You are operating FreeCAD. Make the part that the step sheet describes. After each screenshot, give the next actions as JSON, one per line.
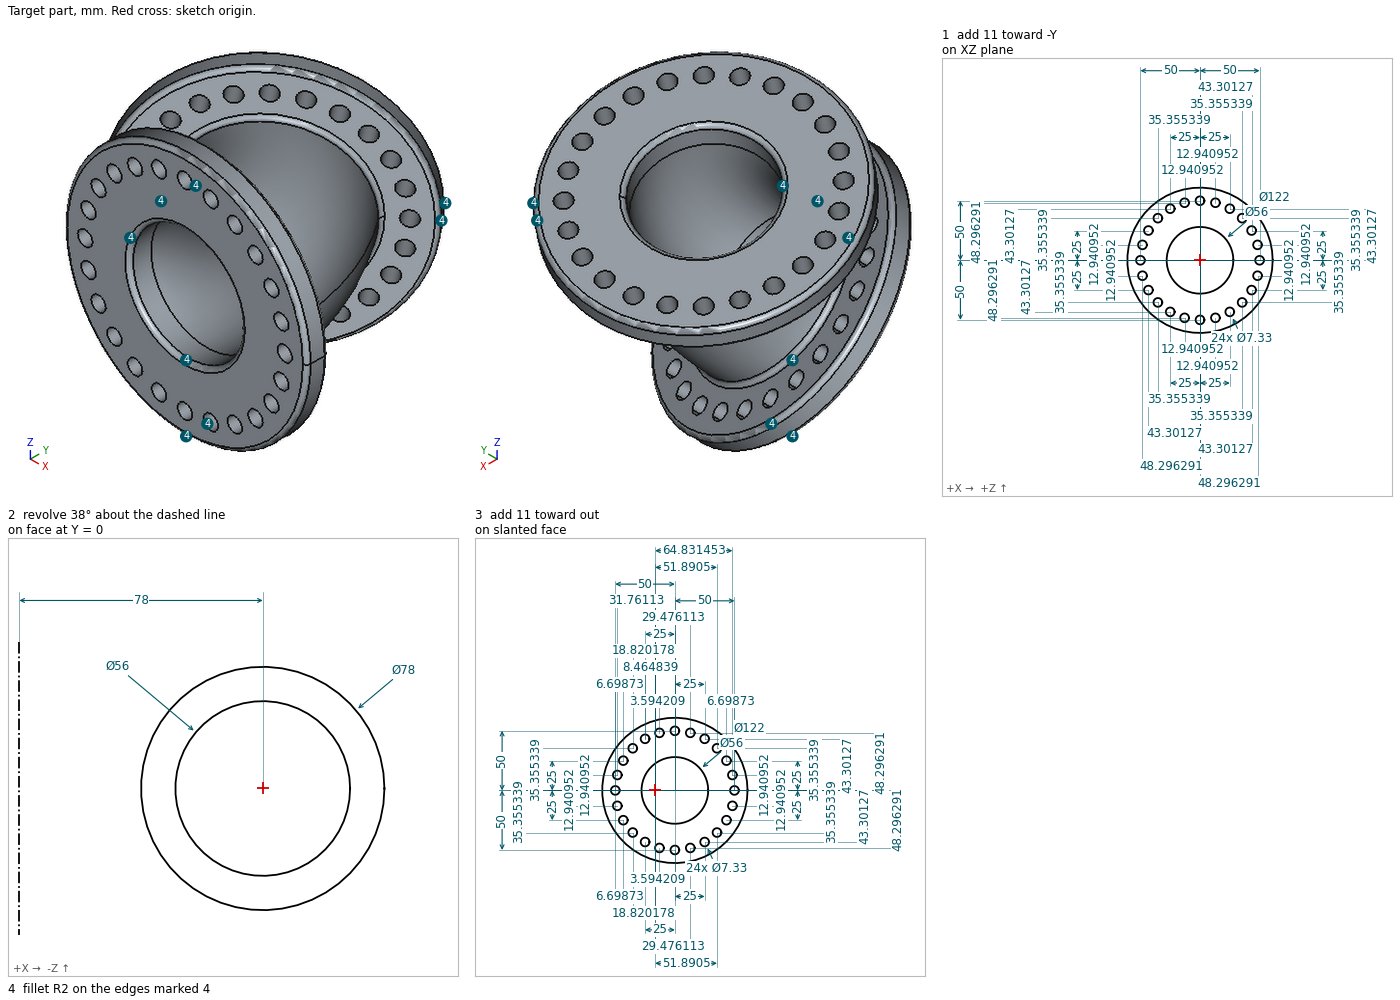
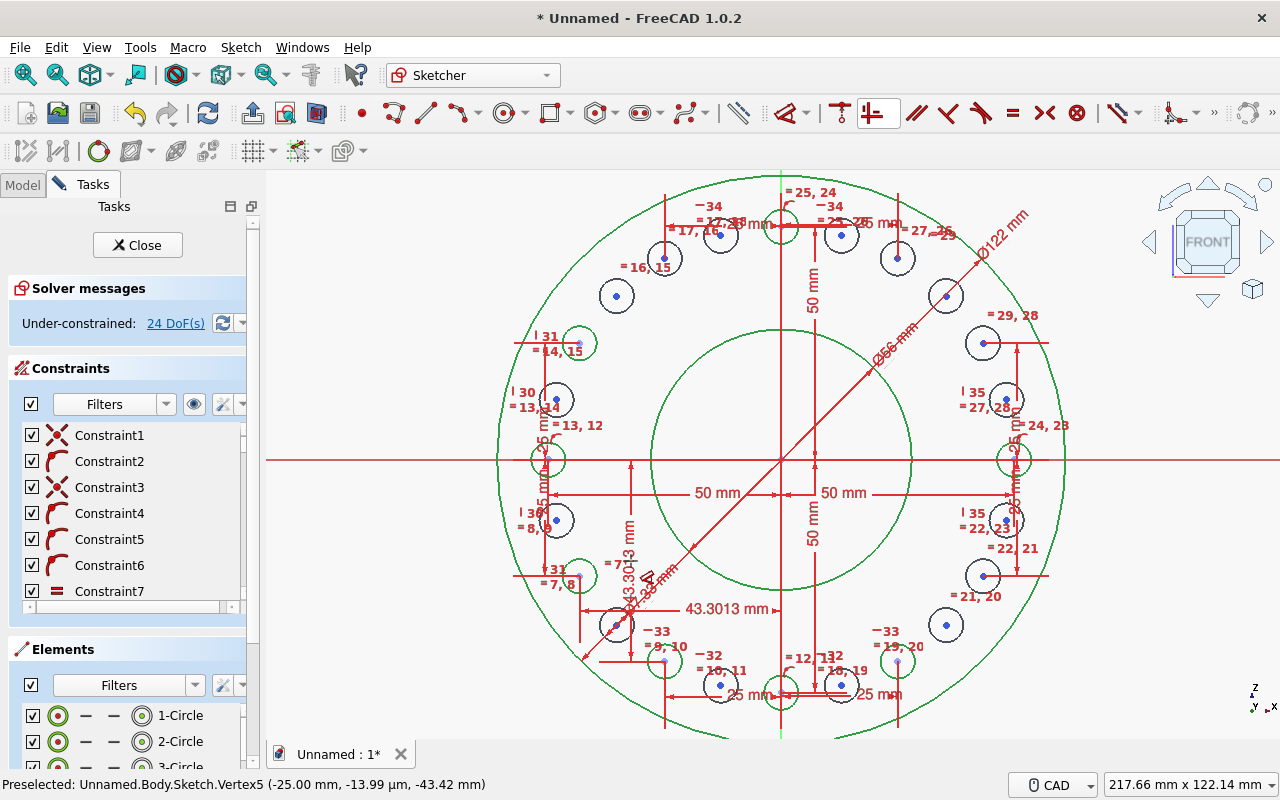
{"action": "left_click", "coordinate": [665, 259]}
{"action": "left_click", "coordinate": [631, 359]}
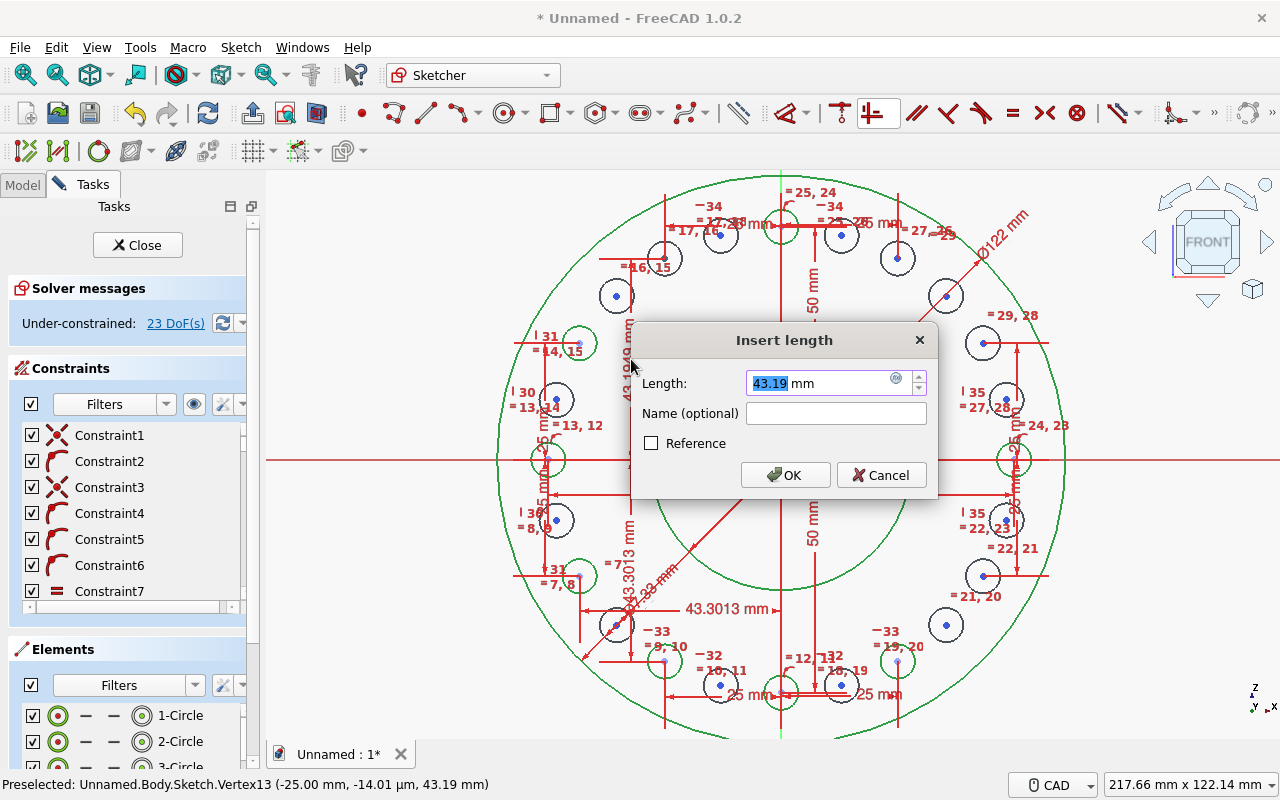
{"action": "type", "text": "43.30127"}
{"action": "key", "text": "Return"}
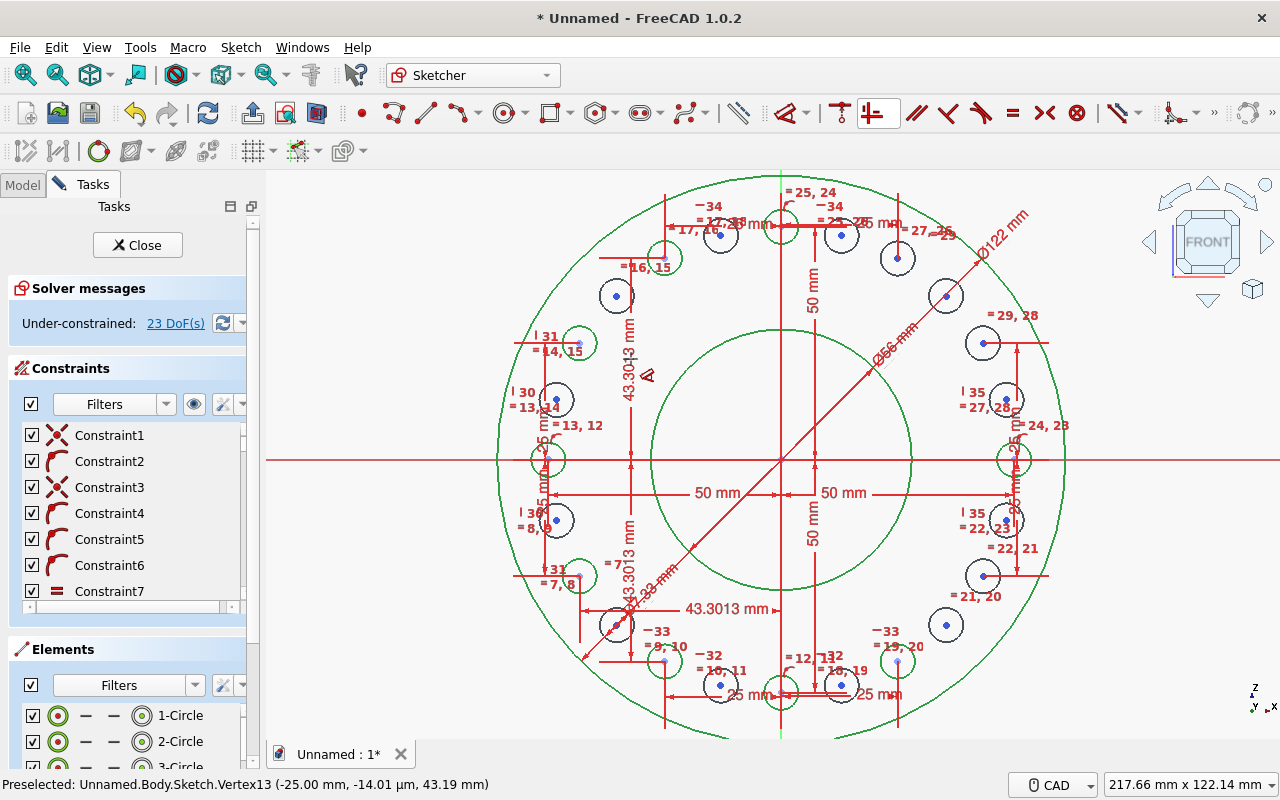
{"action": "left_click", "coordinate": [983, 576]}
{"action": "left_click", "coordinate": [882, 610]}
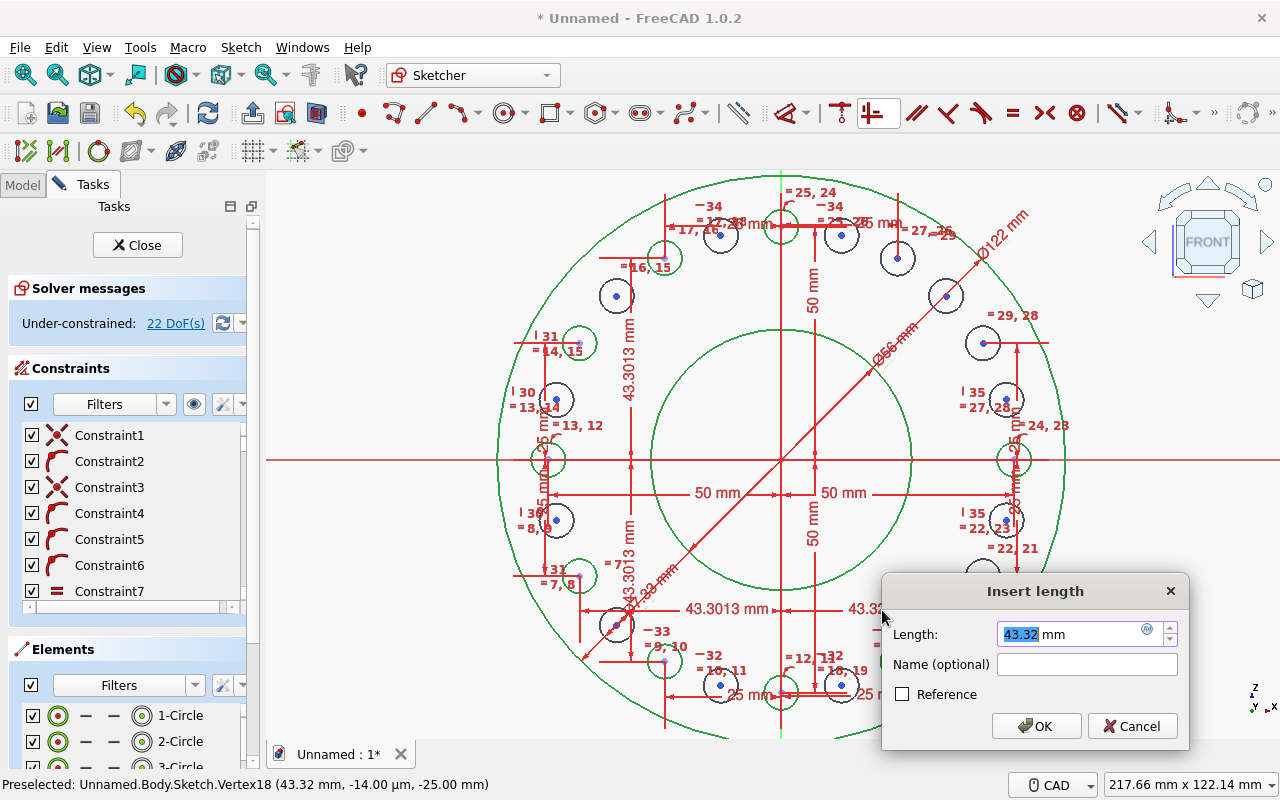
{"action": "type", "text": "43.30127"}
{"action": "key", "text": "Return"}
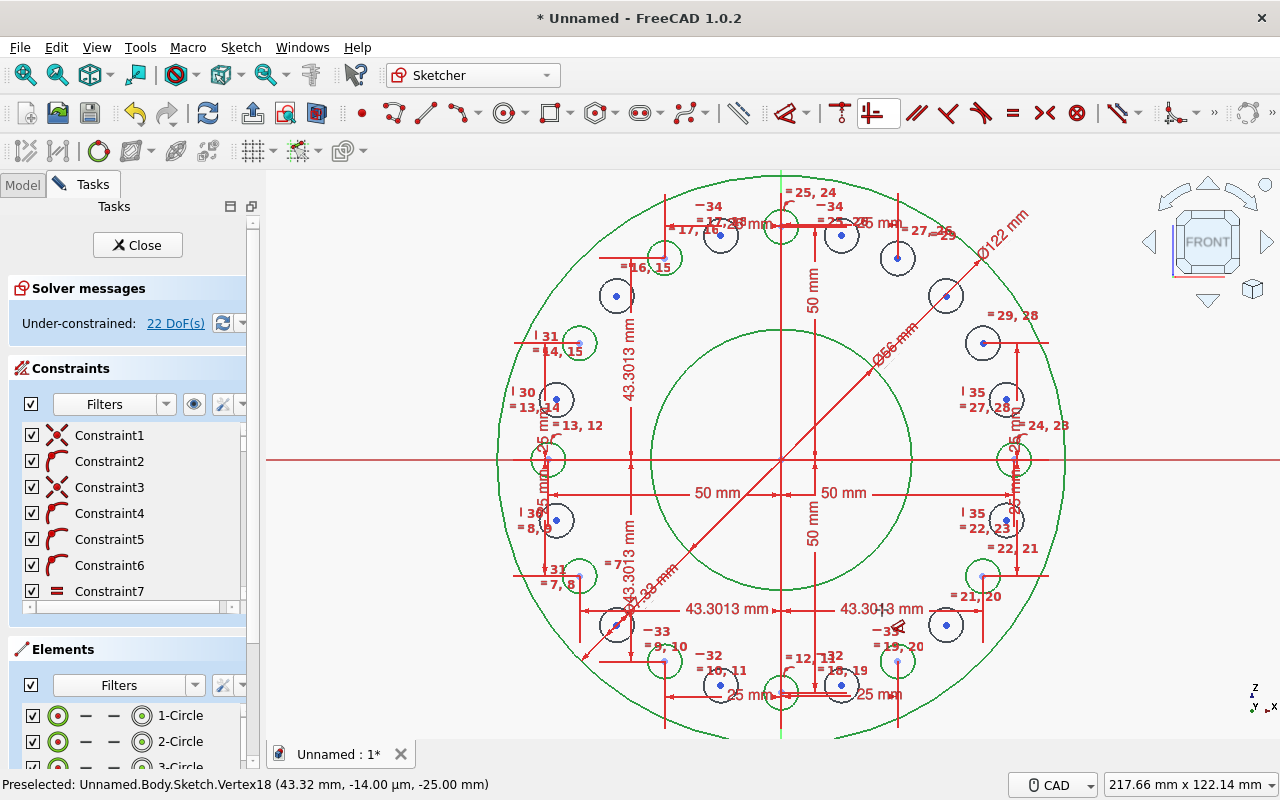
{"action": "left_click", "coordinate": [898, 258]}
{"action": "left_click", "coordinate": [932, 405]}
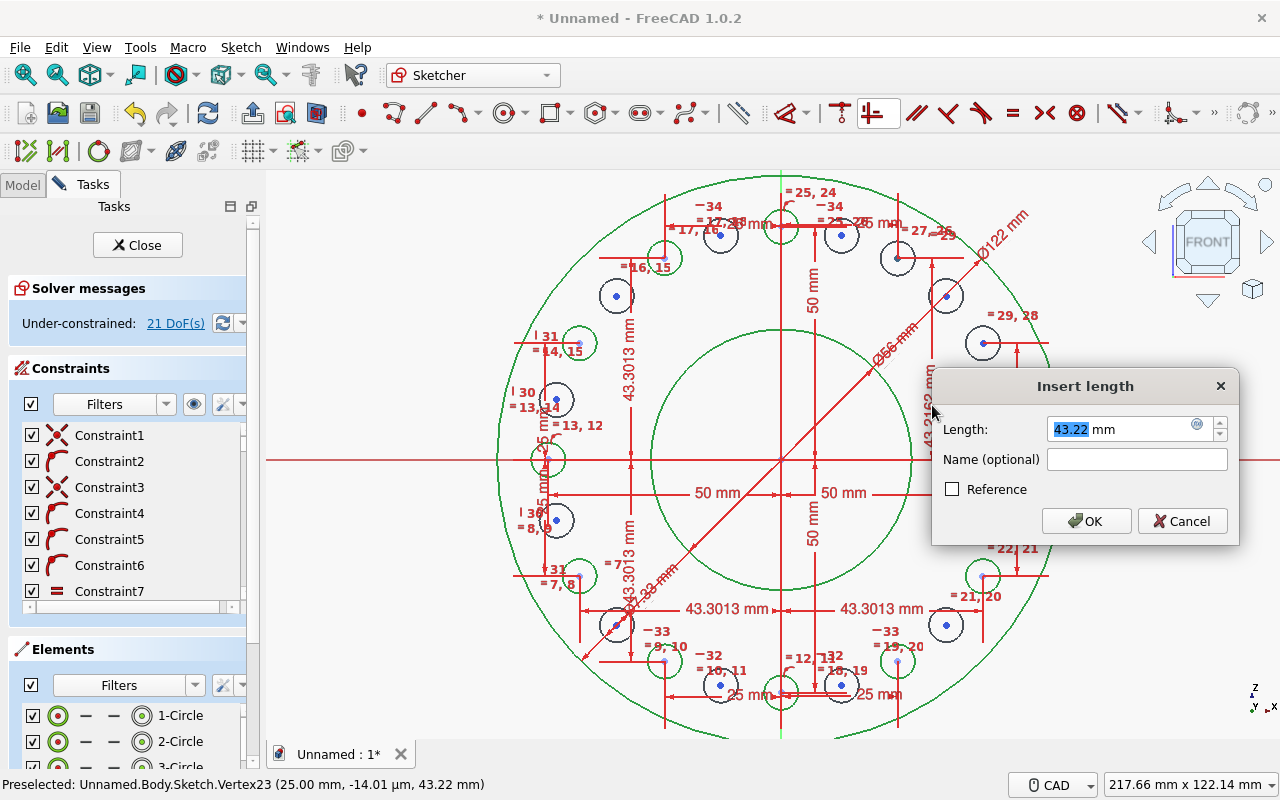
{"action": "type", "text": "43.30127"}
{"action": "key", "text": "Return"}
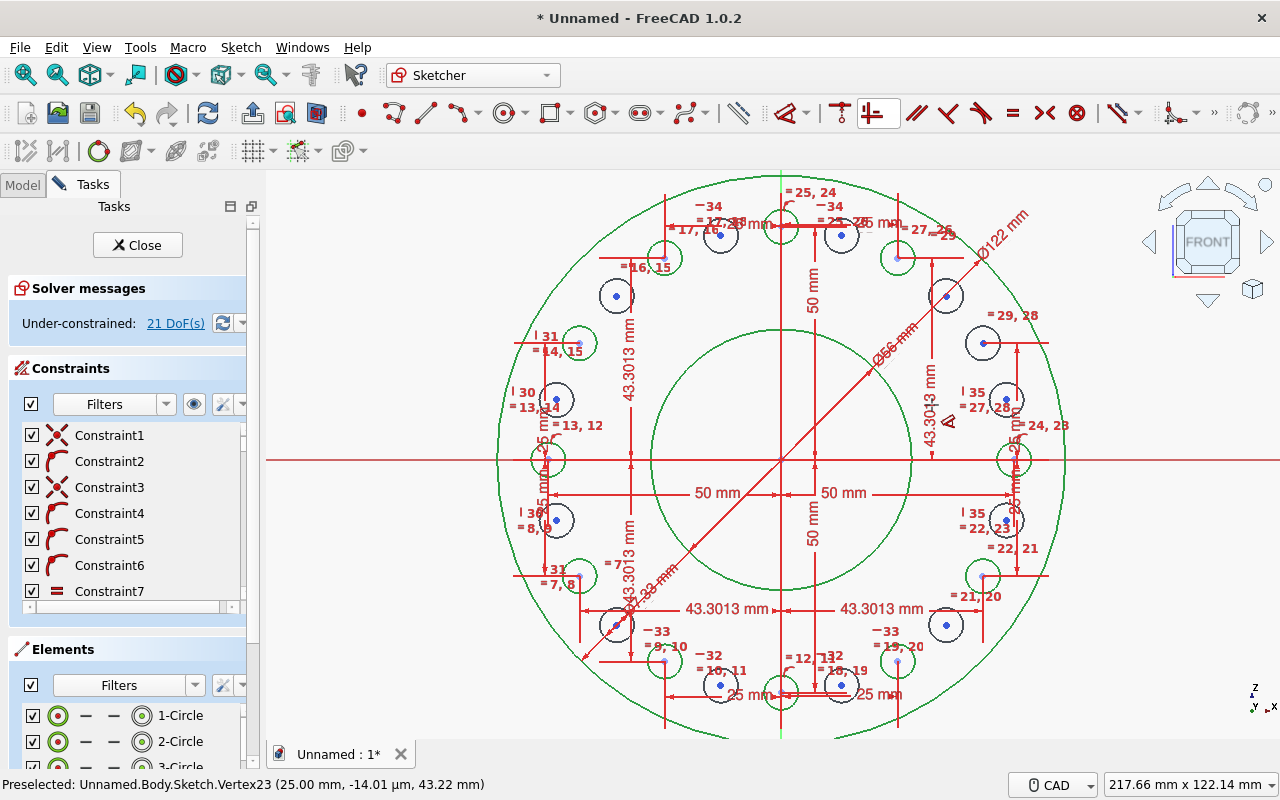
{"action": "left_click", "coordinate": [983, 343]}
{"action": "left_click", "coordinate": [929, 494]}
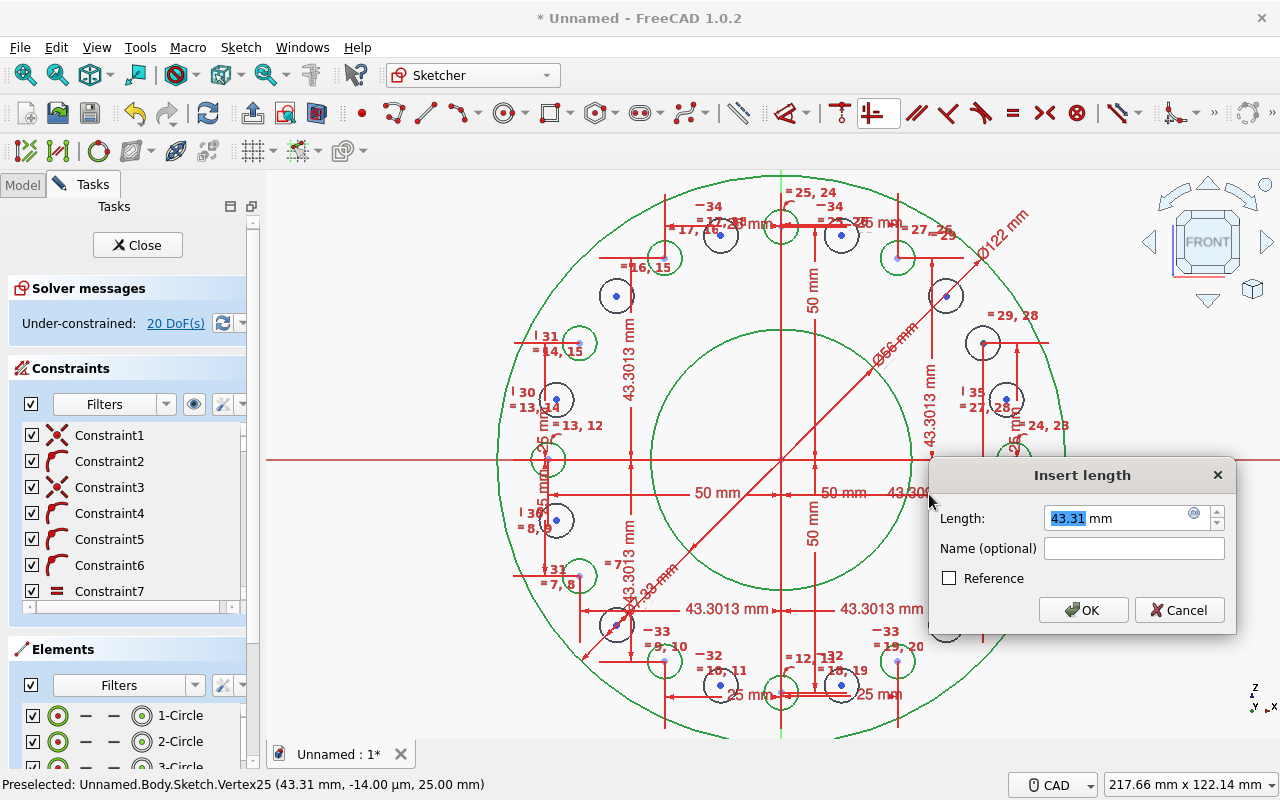
{"action": "type", "text": "43.30127"}
{"action": "key", "text": "Return"}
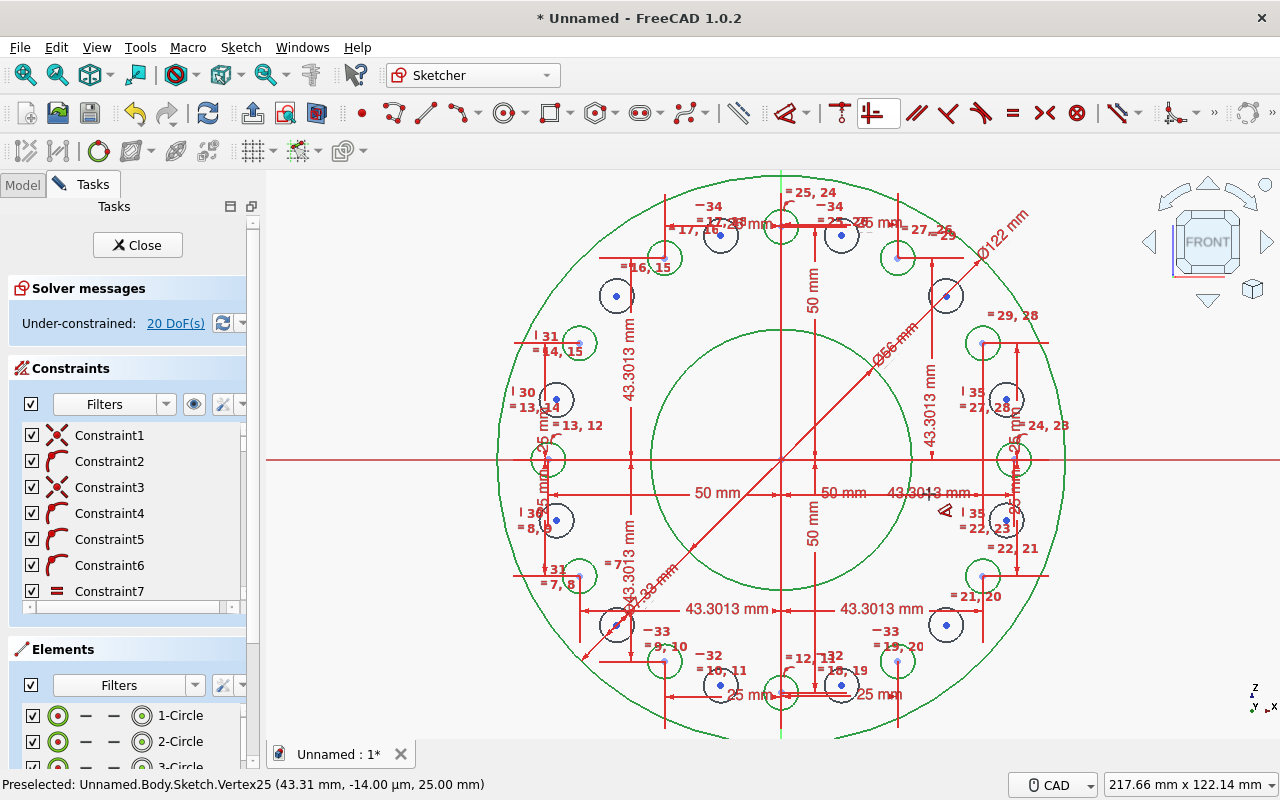
{"action": "left_click", "coordinate": [617, 625]}
{"action": "left_click", "coordinate": [699, 659]}